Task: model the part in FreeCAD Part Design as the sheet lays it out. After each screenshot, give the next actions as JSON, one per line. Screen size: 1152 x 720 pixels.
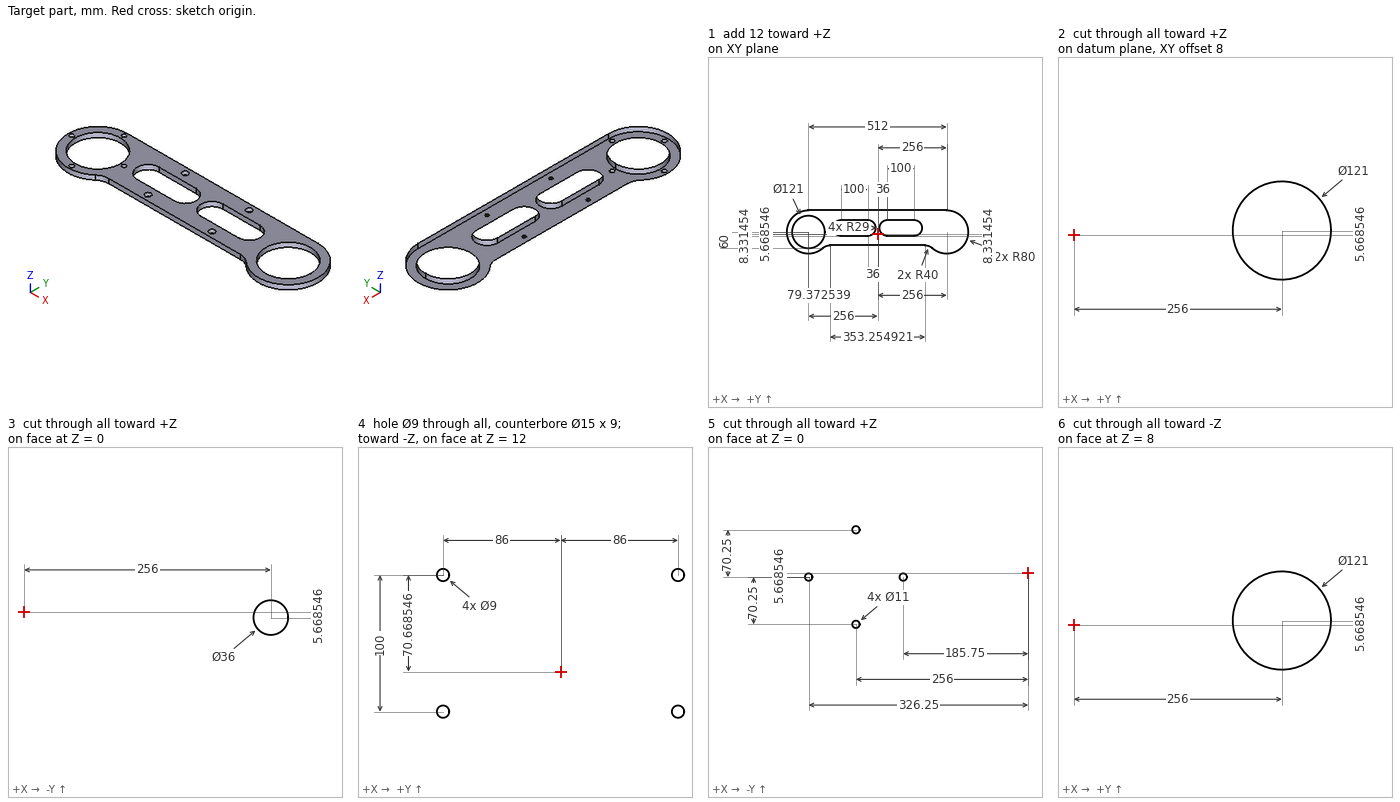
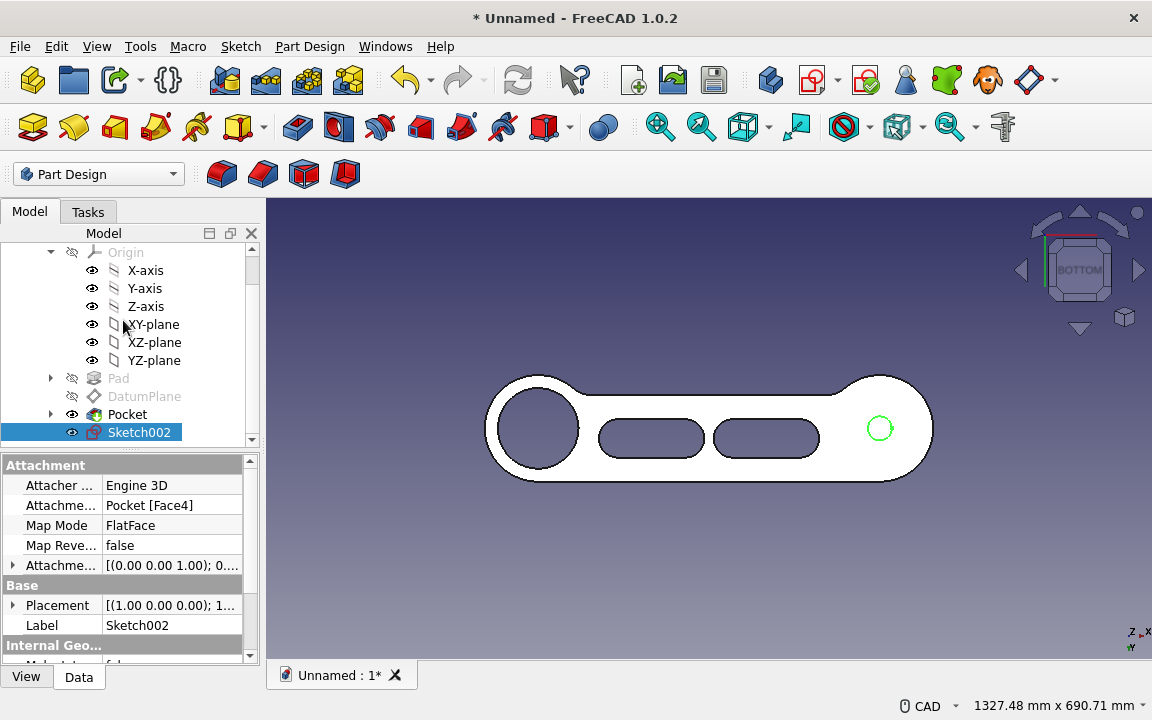
{"action": "left_click", "coordinate": [298, 128]}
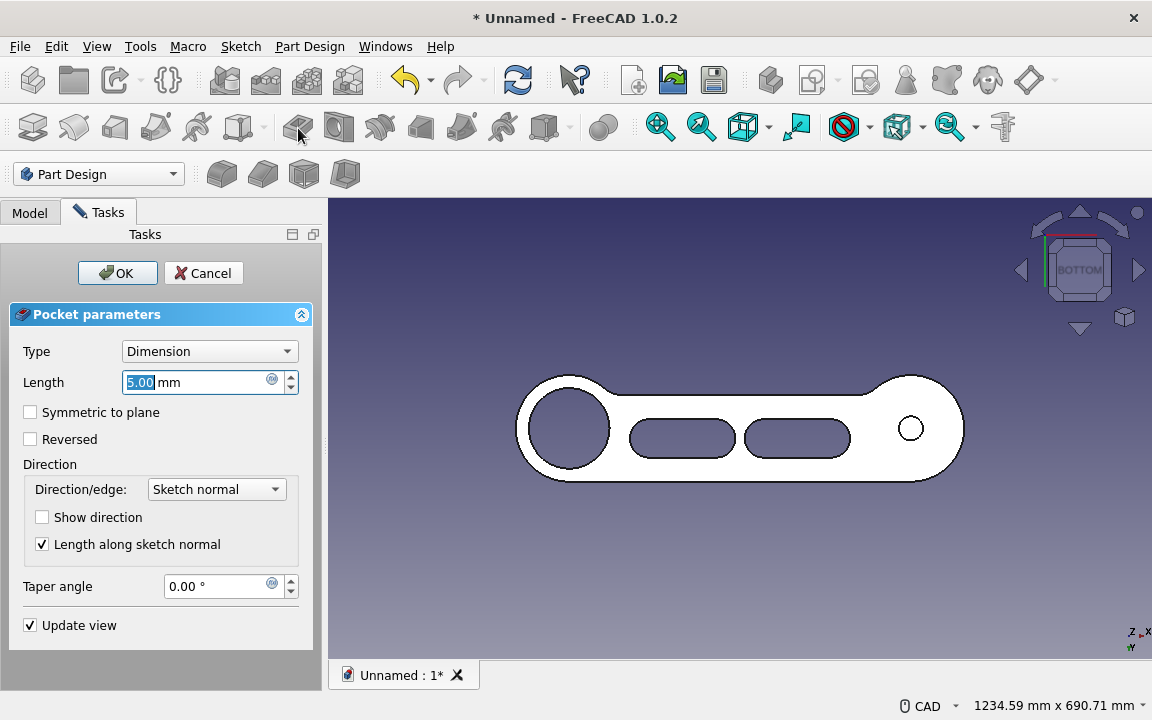
{"action": "left_click", "coordinate": [210, 352]}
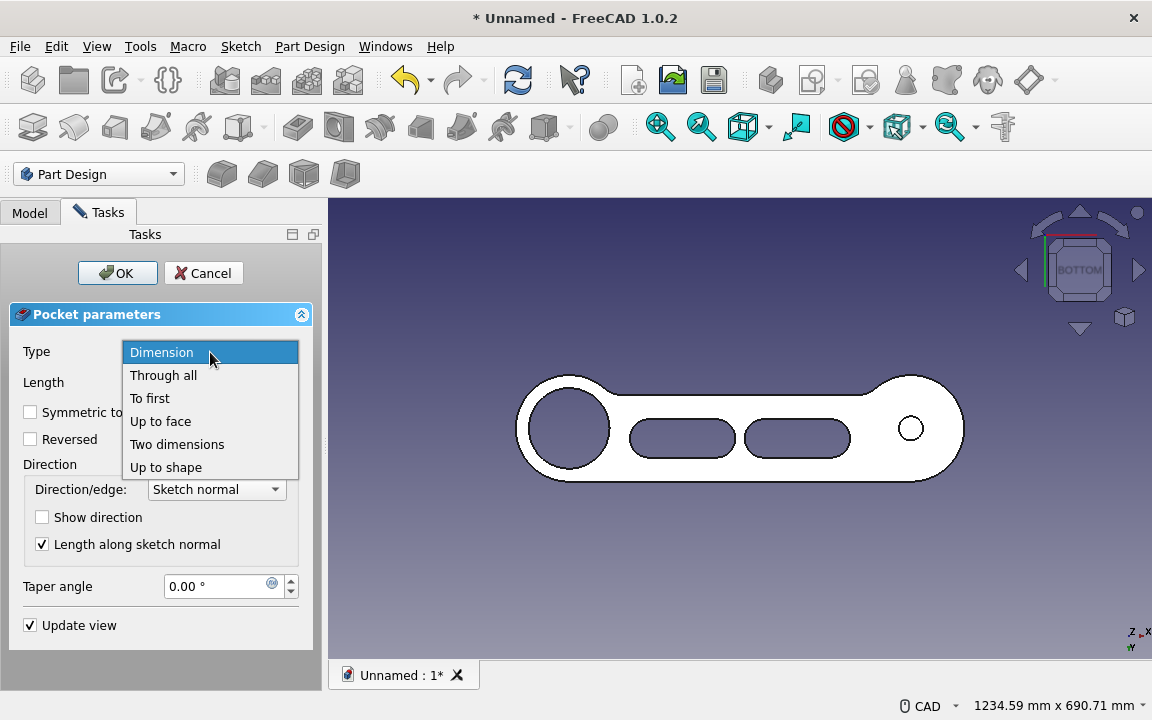
{"action": "left_click", "coordinate": [208, 376]}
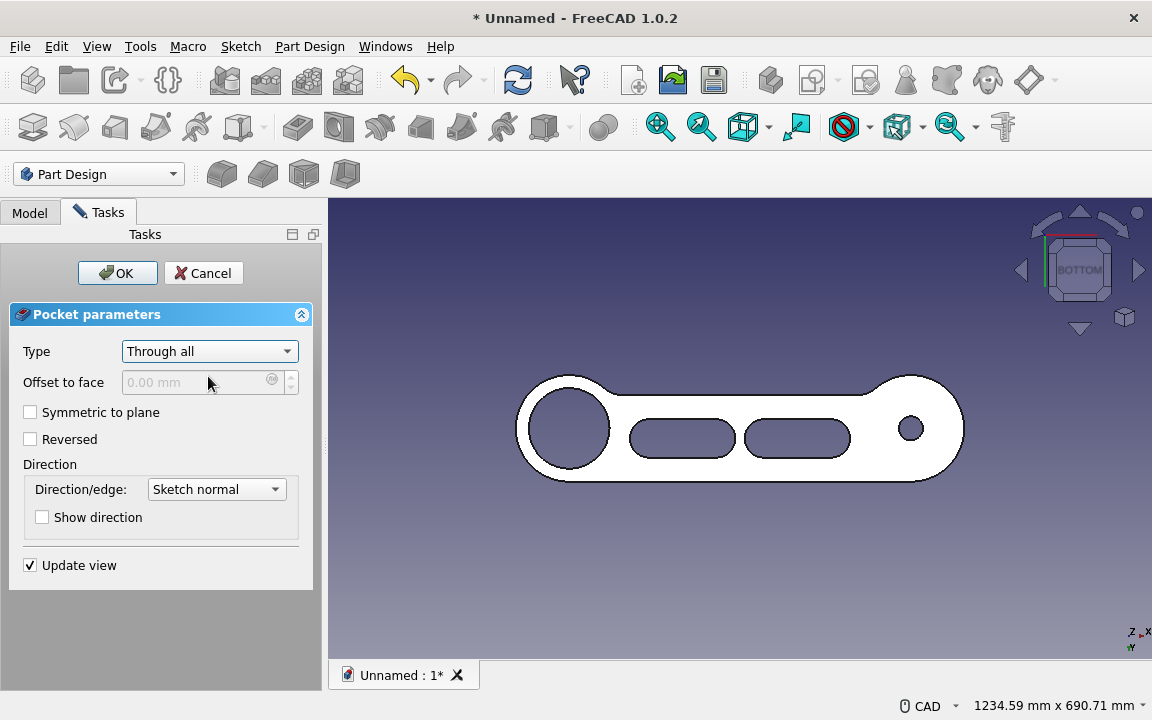
{"action": "left_click", "coordinate": [118, 273]}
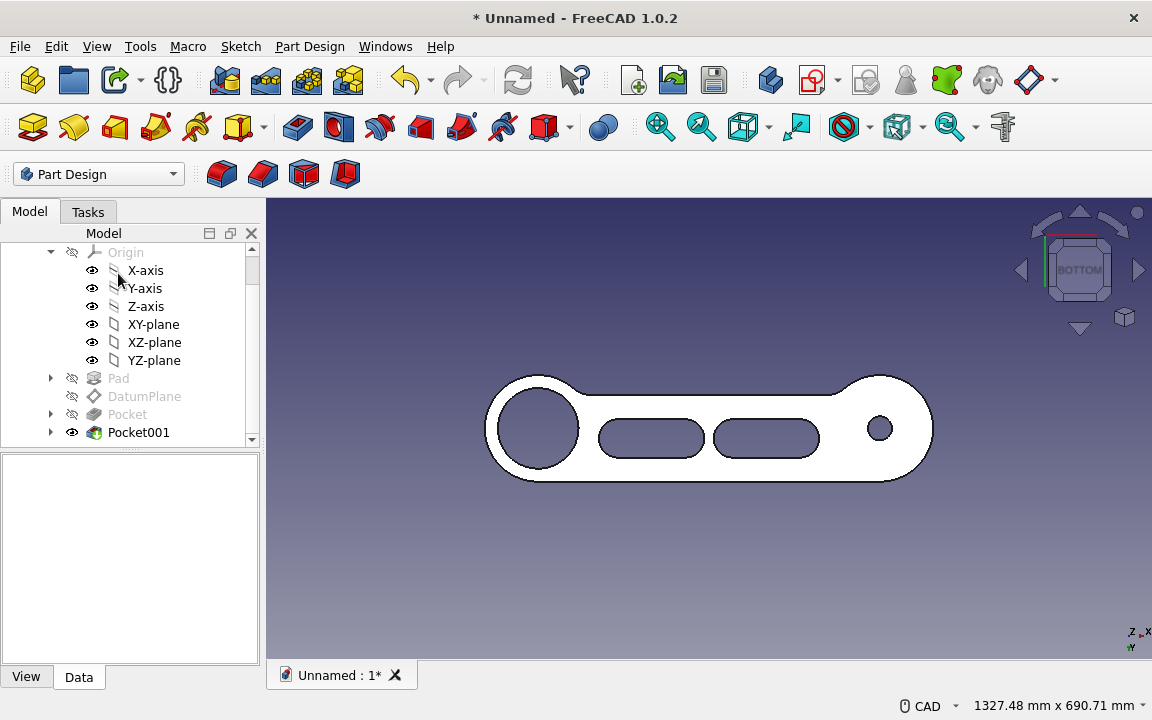
{"action": "key", "text": "0"}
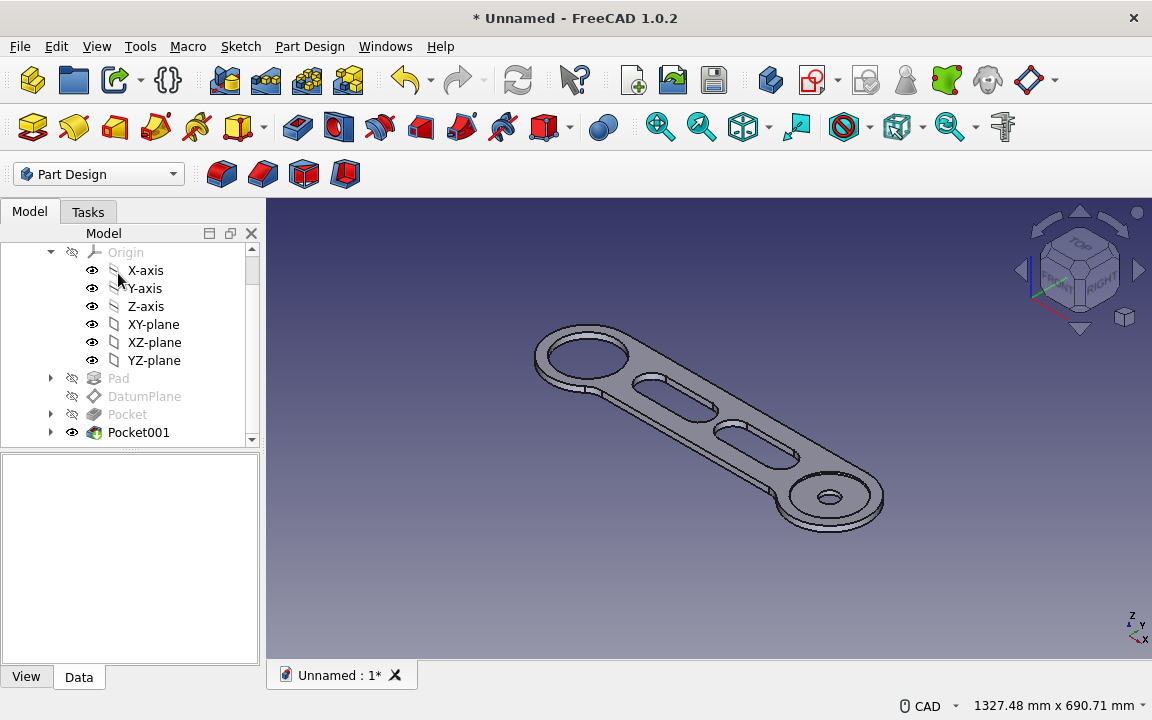
{"action": "left_click", "coordinate": [698, 430]}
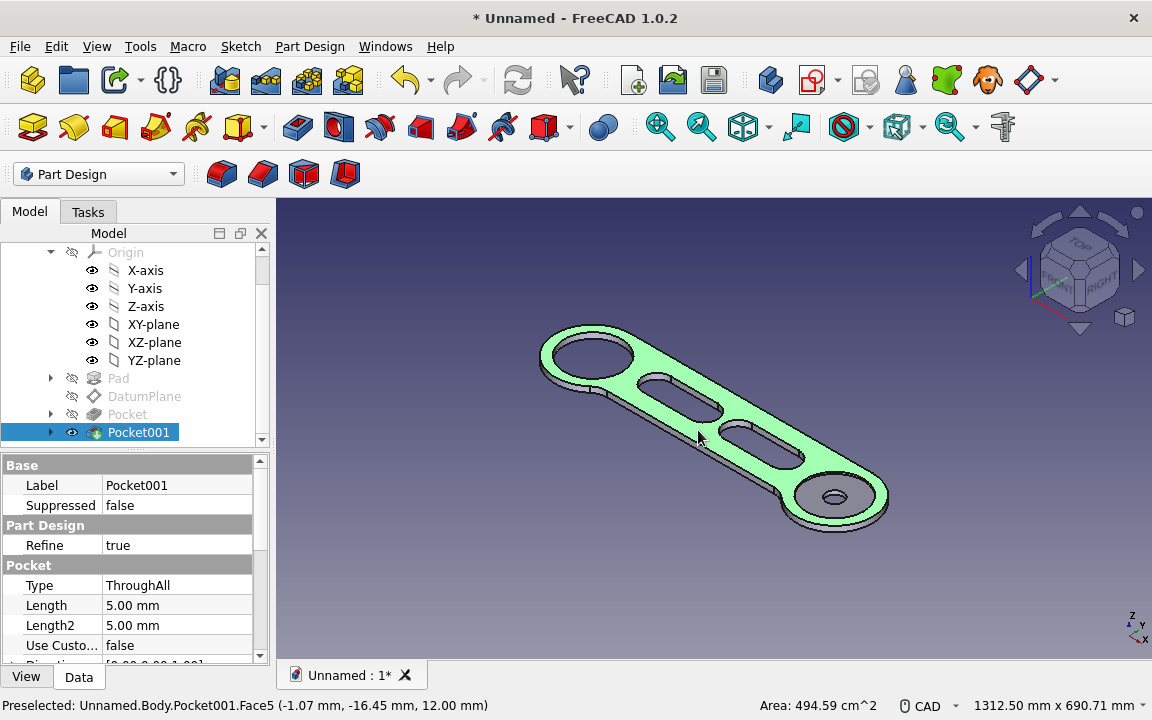
{"action": "left_click", "coordinate": [812, 80]}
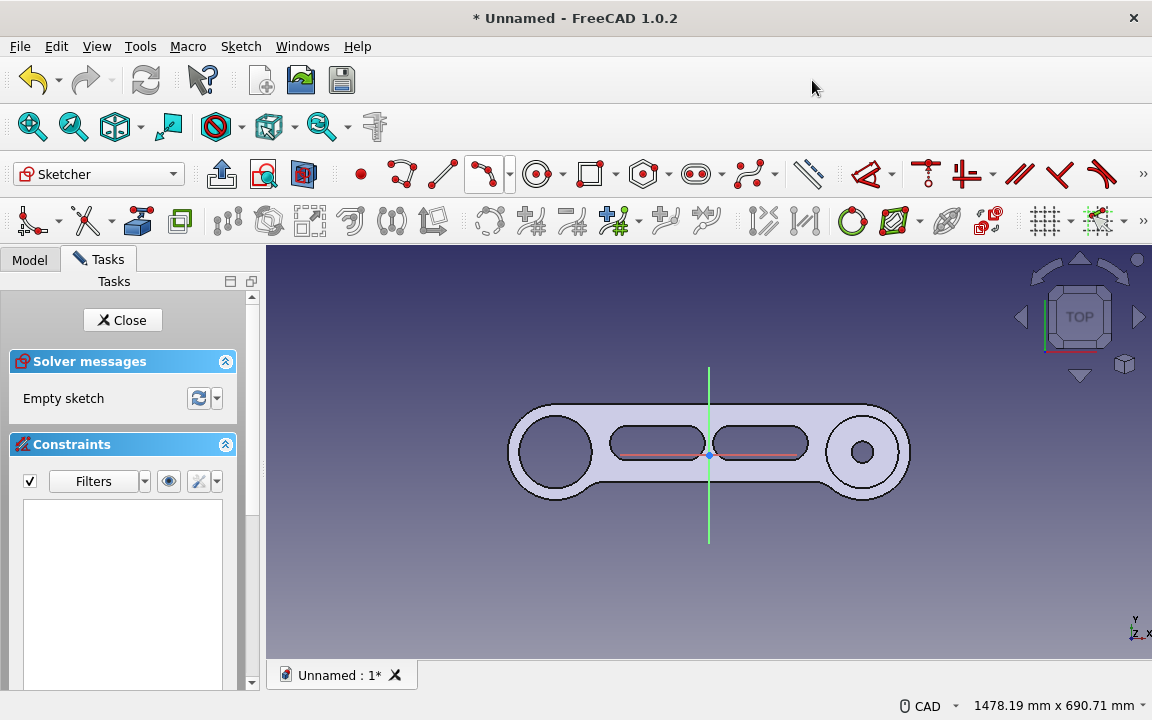
{"action": "scroll", "coordinate": [731, 440], "scroll_direction": "up", "scroll_amount": 7}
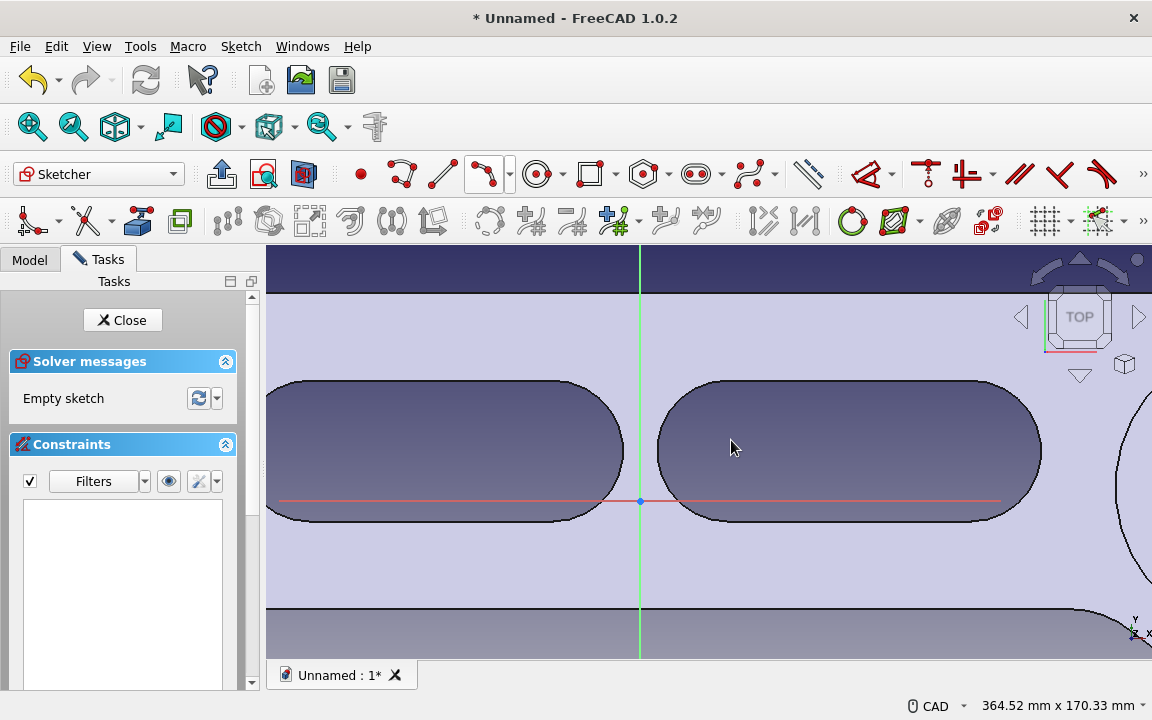
{"action": "left_click", "coordinate": [536, 174]}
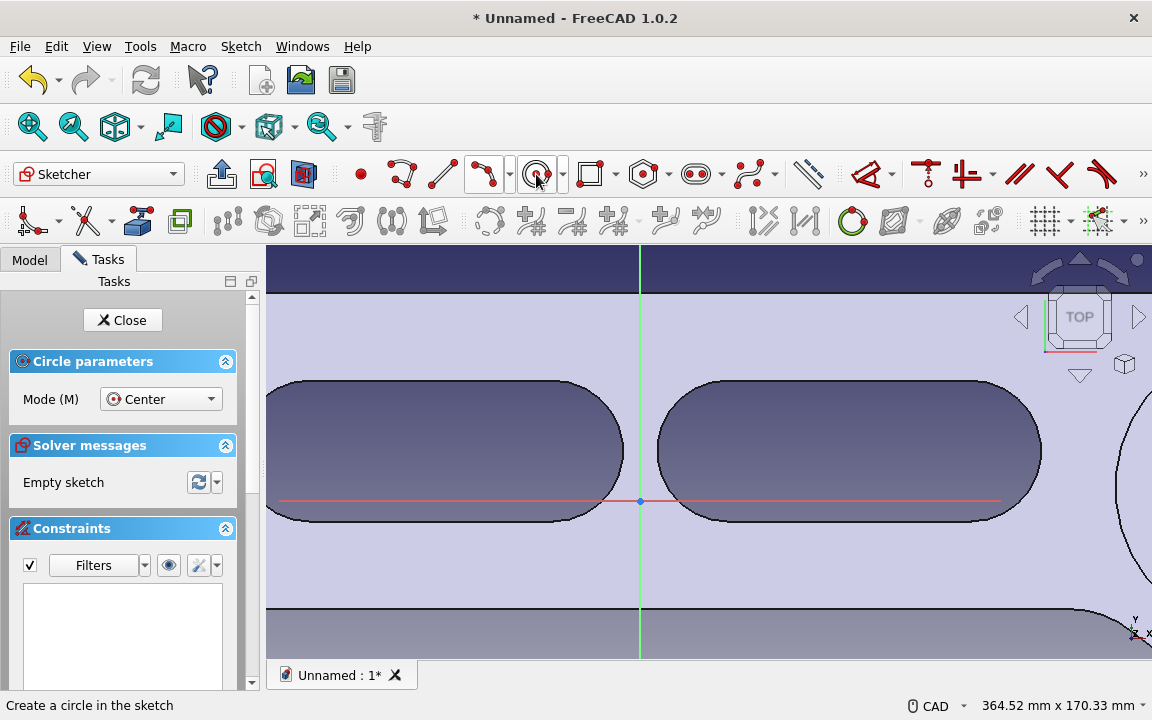
{"action": "scroll", "coordinate": [431, 330], "scroll_direction": "up", "scroll_amount": 4}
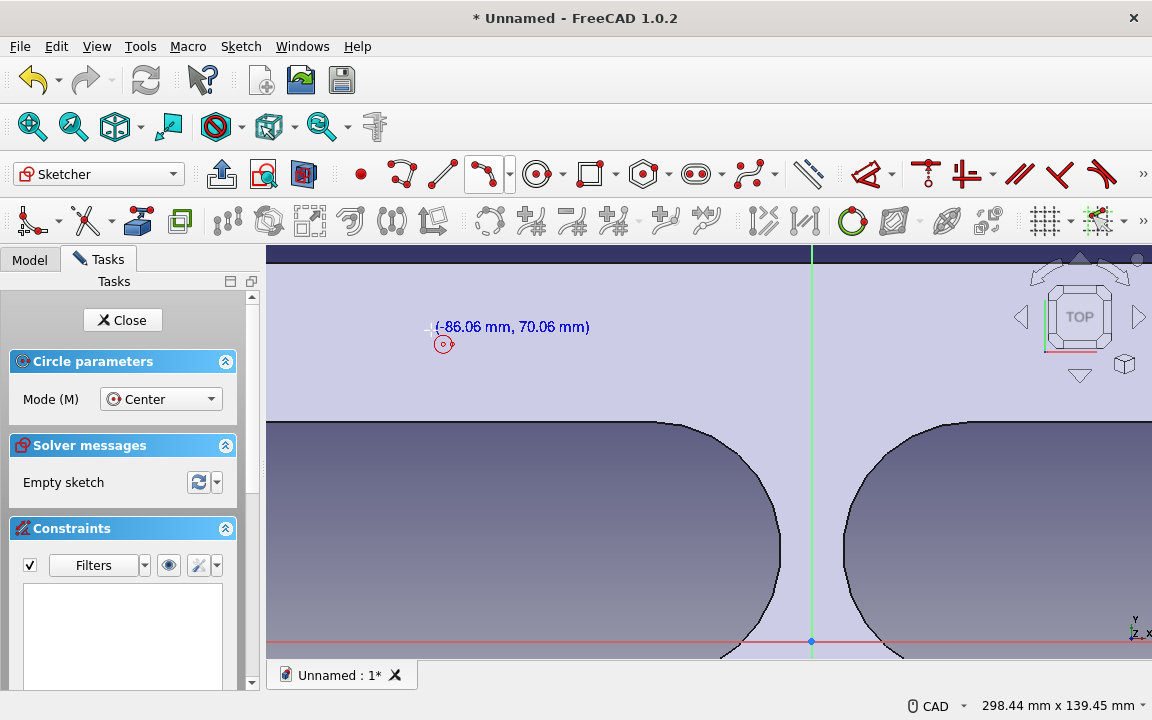
{"action": "left_click", "coordinate": [431, 329]}
{"action": "mouse_move", "coordinate": [448, 311]}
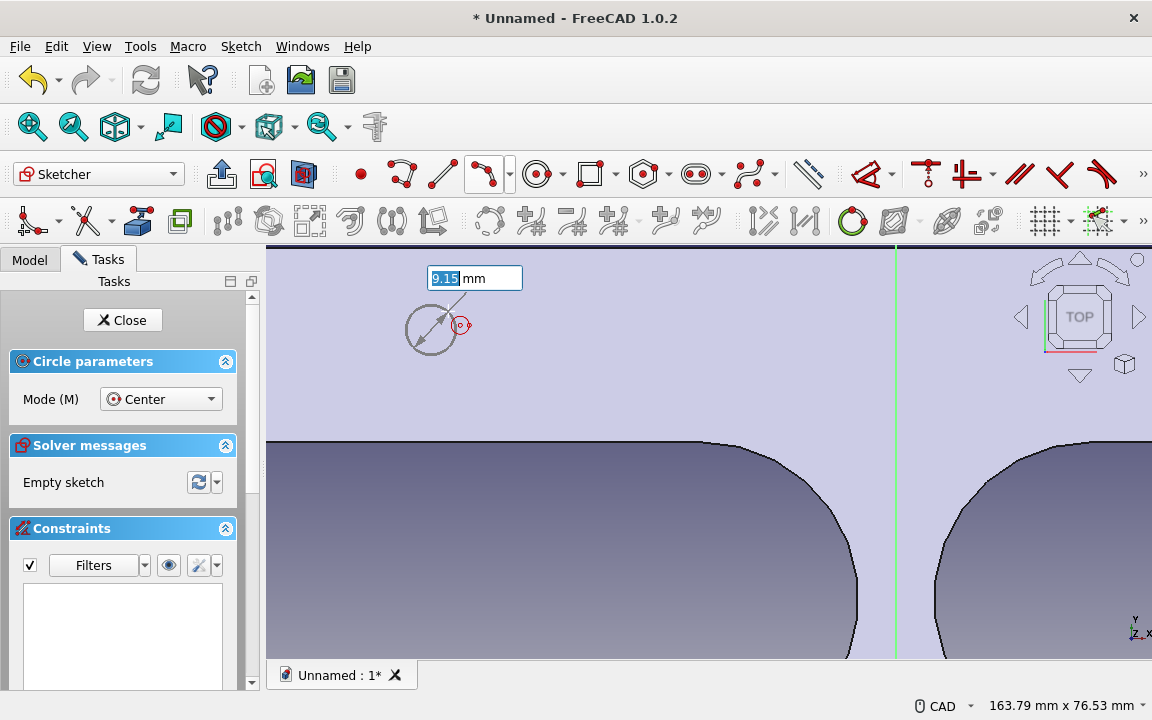
{"action": "type", "text": "9"}
{"action": "key", "text": "Return"}